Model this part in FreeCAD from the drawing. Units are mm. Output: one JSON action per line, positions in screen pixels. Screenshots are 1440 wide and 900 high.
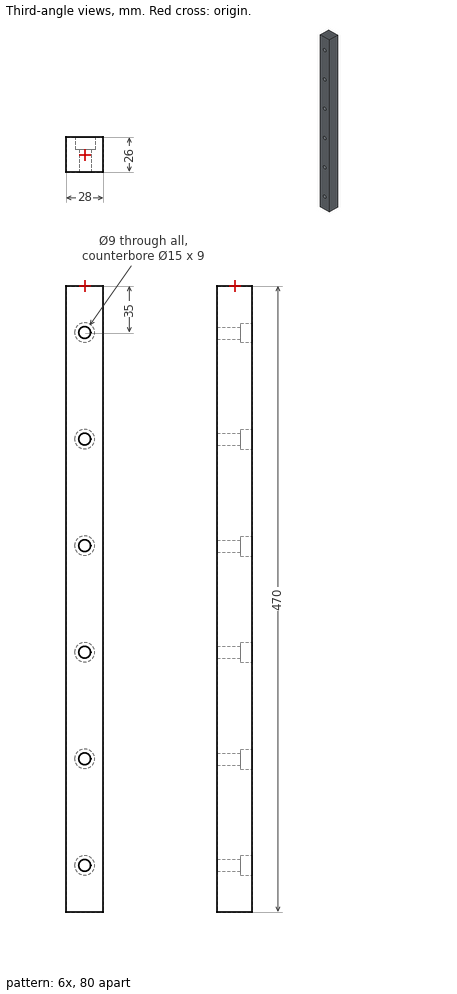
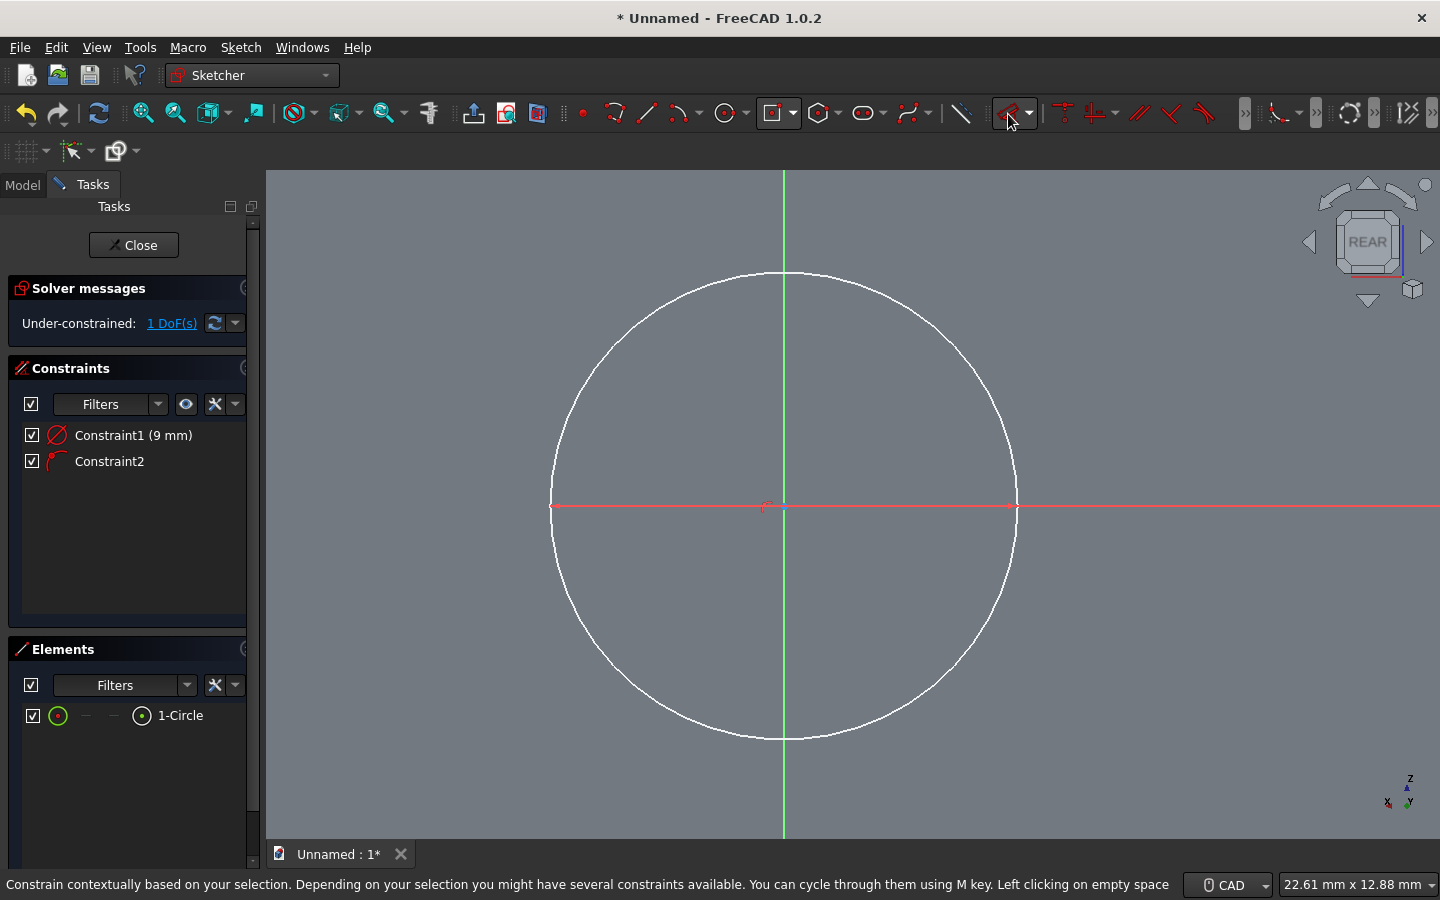
{"action": "left_click", "coordinate": [784, 506]}
{"action": "left_click", "coordinate": [818, 352]}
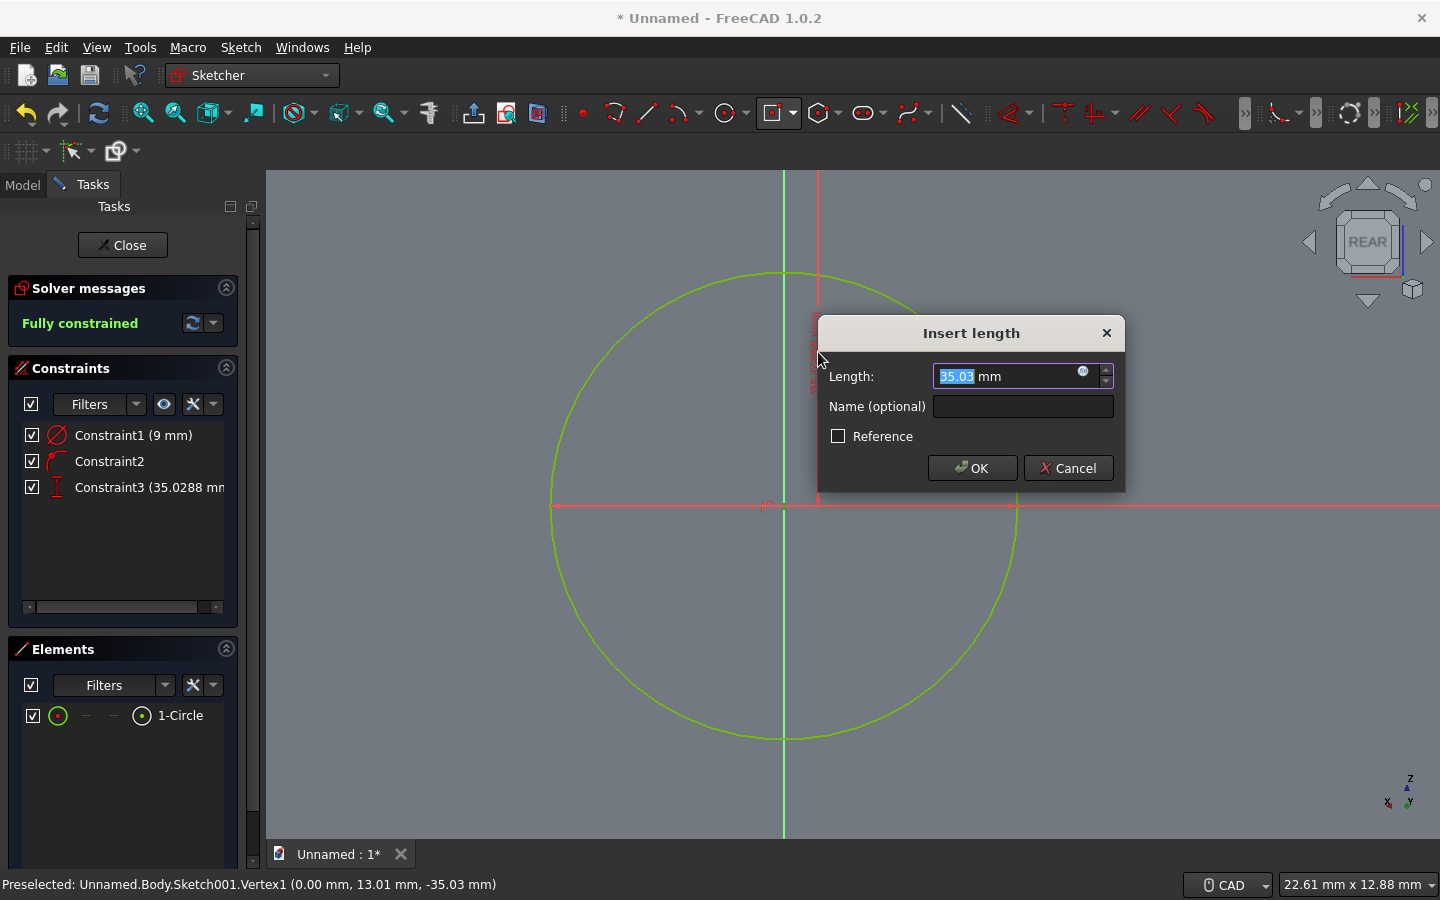
{"action": "type", "text": "35"}
{"action": "key", "text": "Return"}
{"action": "key", "text": "Escape"}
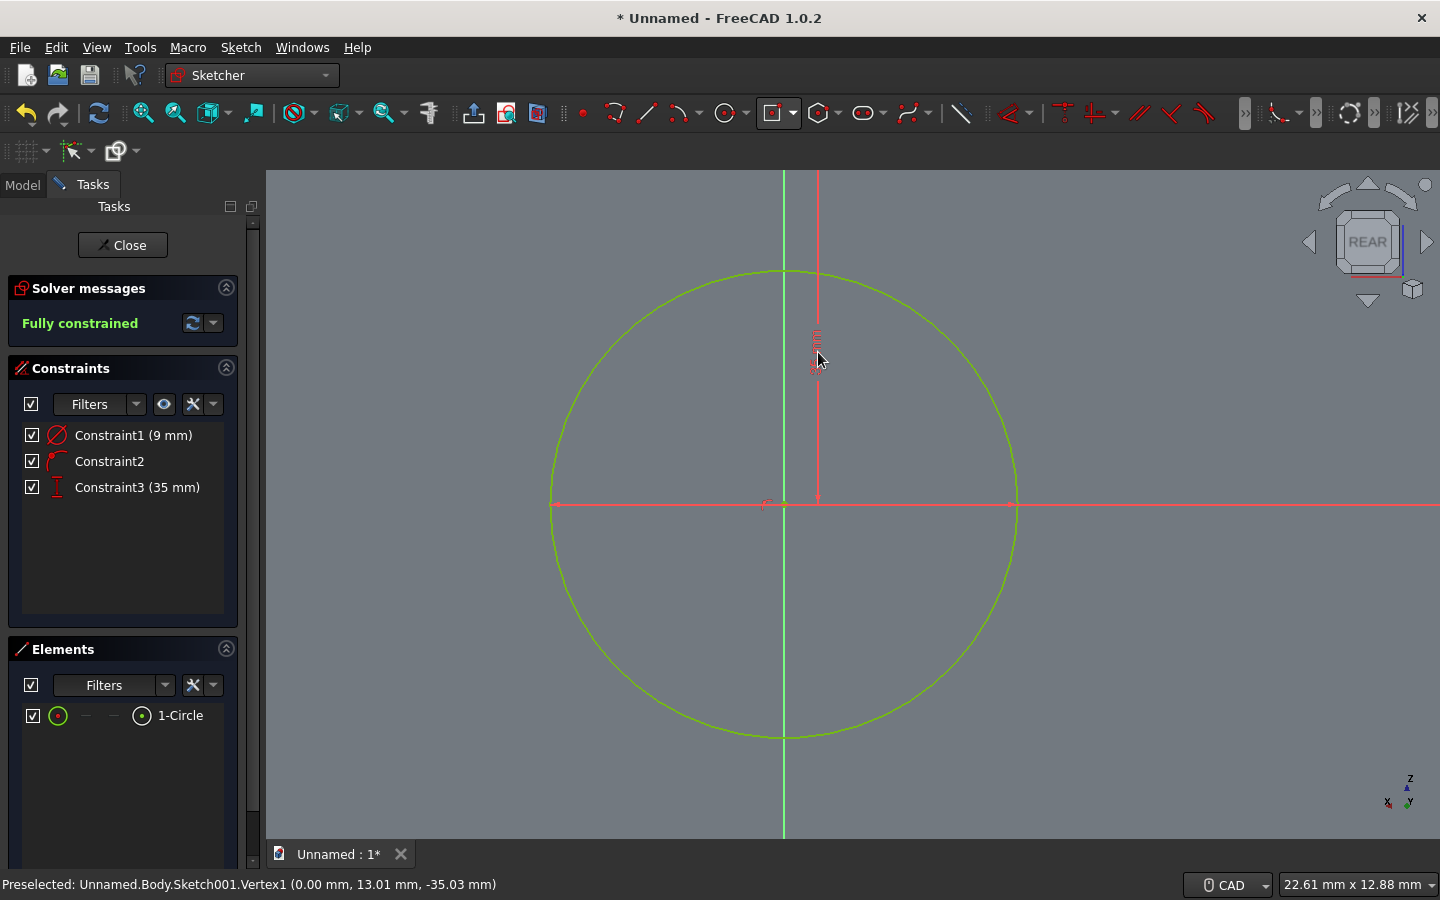
{"action": "left_click", "coordinate": [123, 245]}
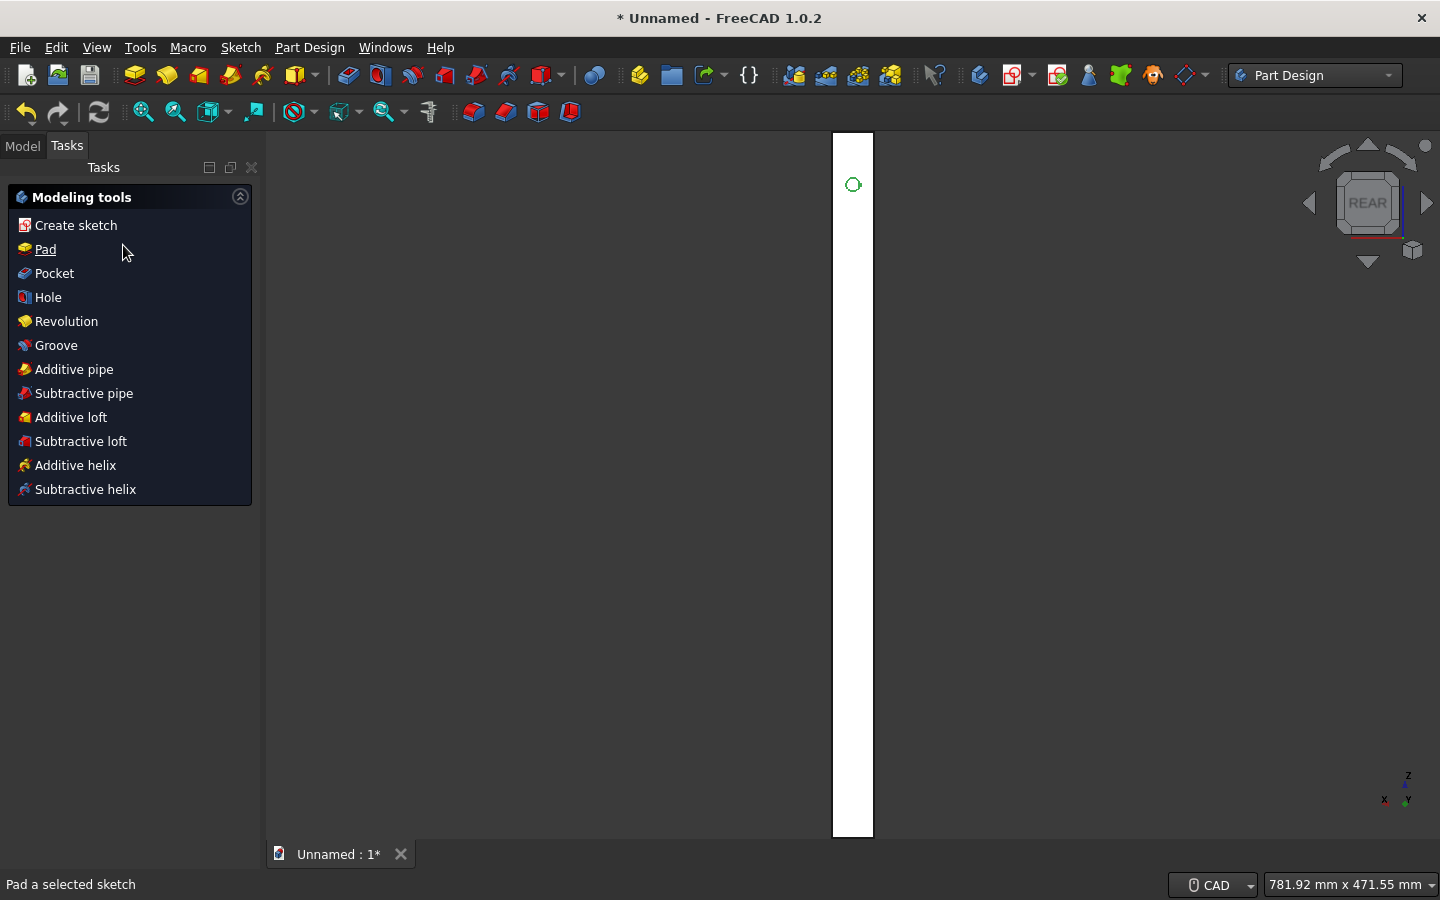
{"action": "left_click", "coordinate": [382, 76]}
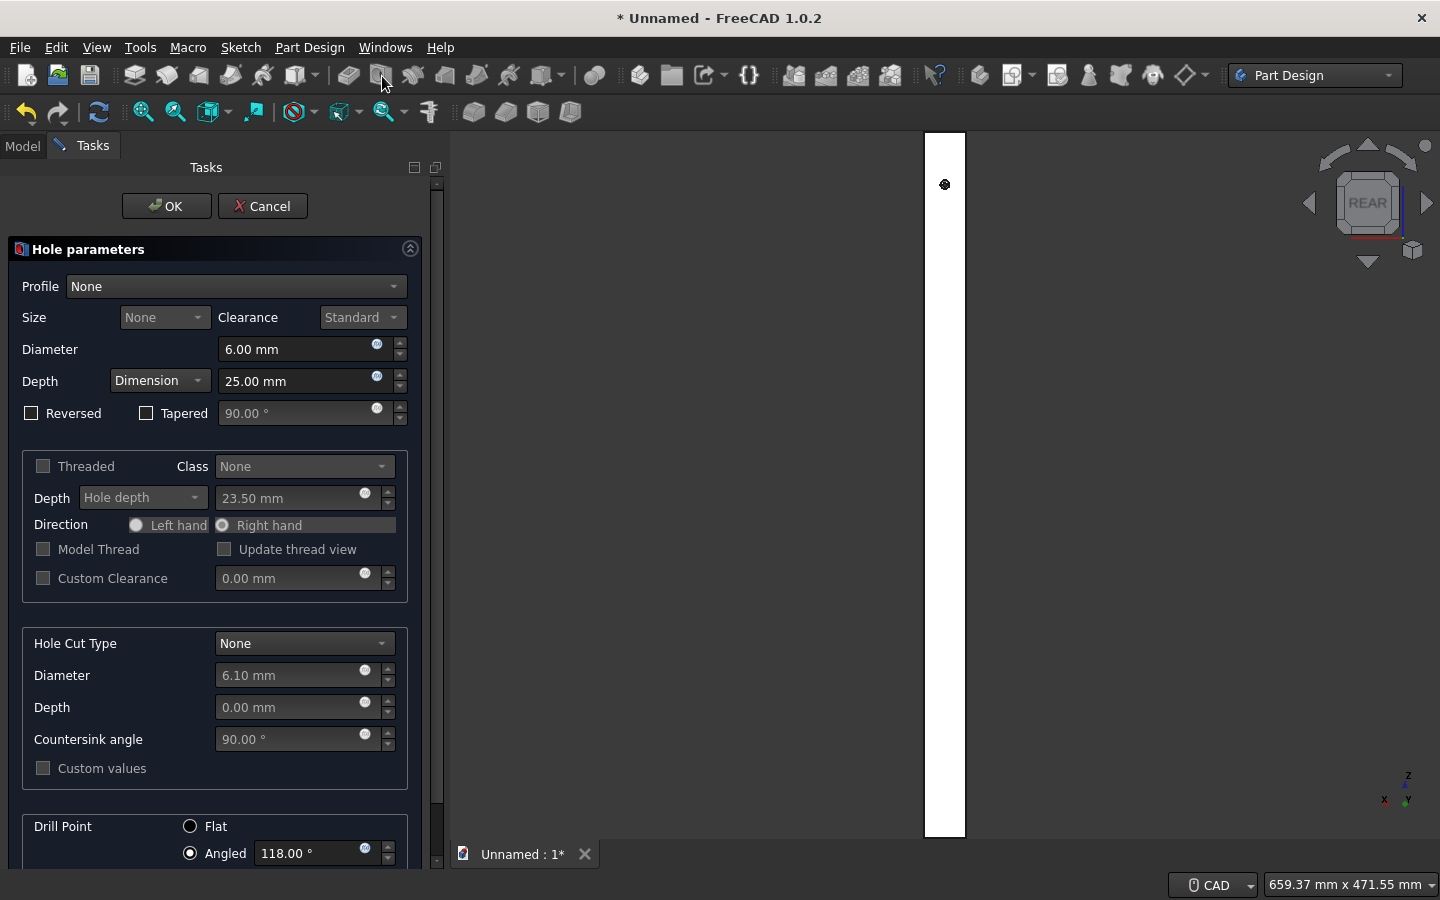
{"action": "triple_click", "coordinate": [305, 349]}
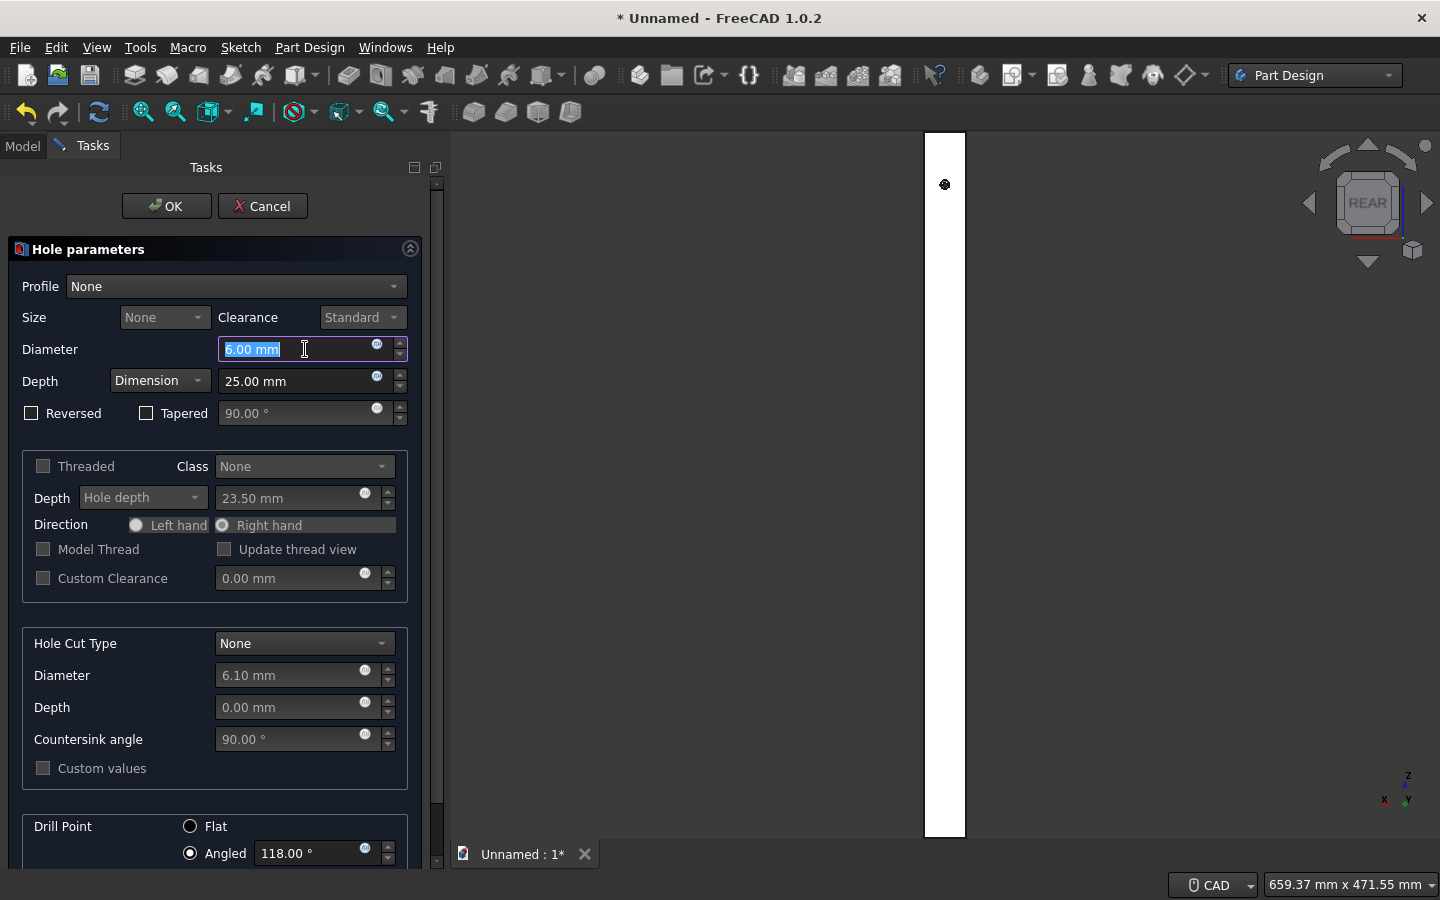
{"action": "type", "text": "9"}
{"action": "key", "text": "Tab"}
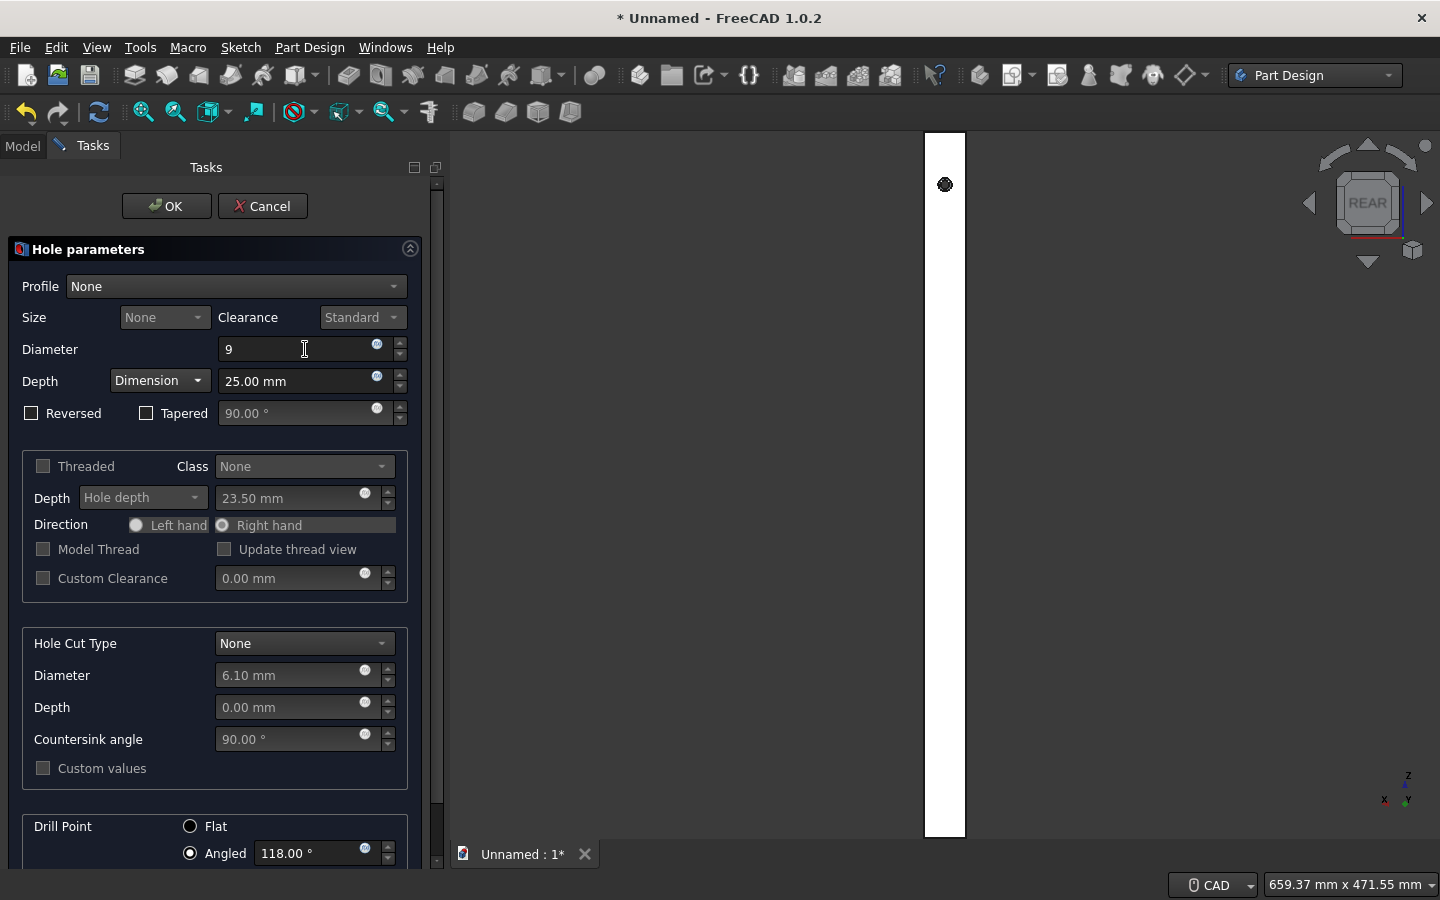
{"action": "left_click", "coordinate": [161, 380]}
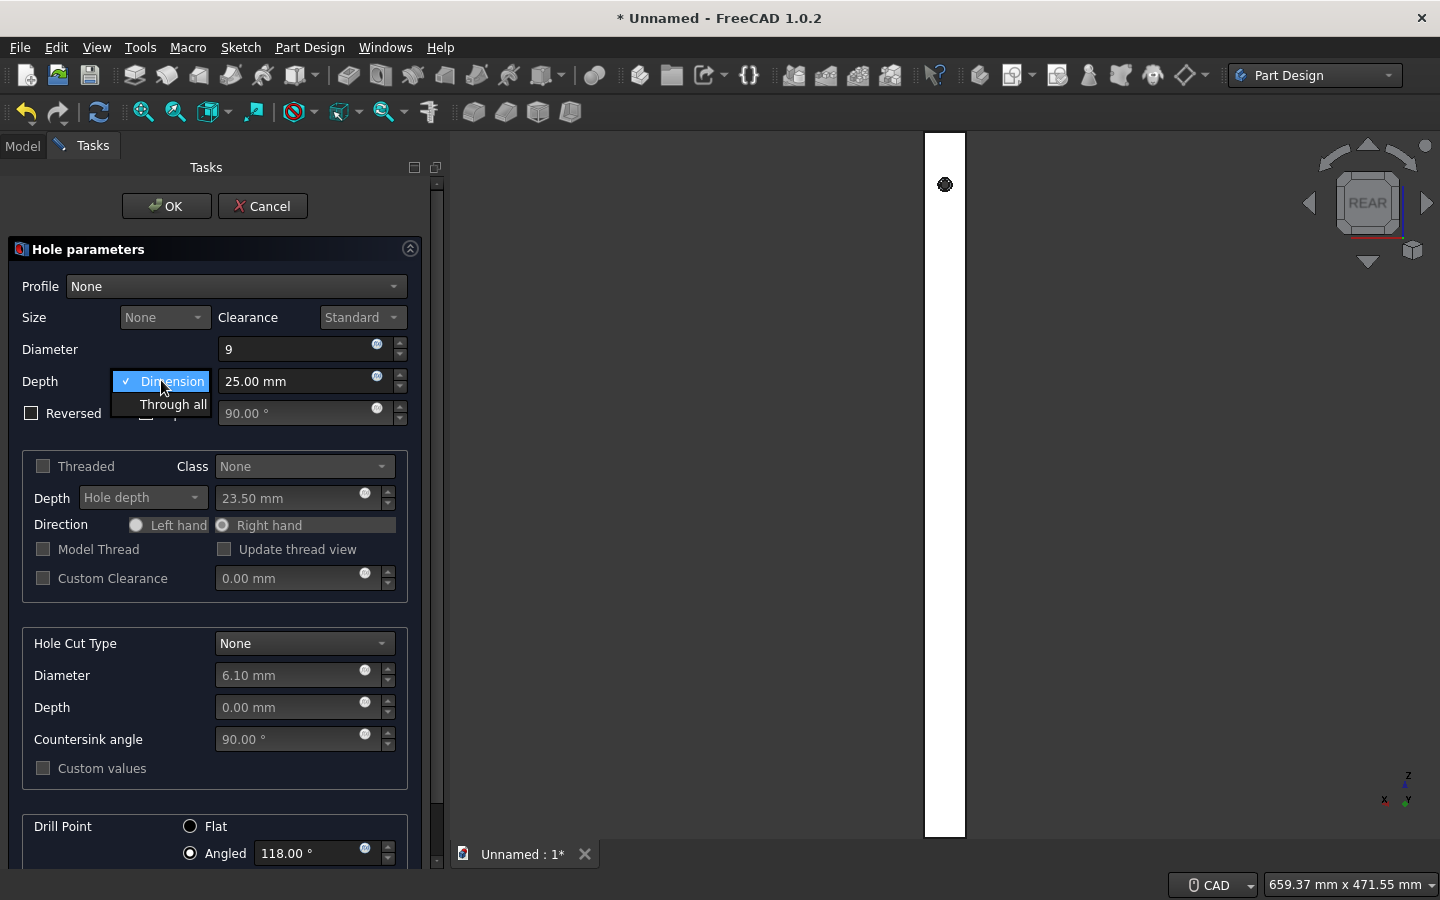
{"action": "left_click", "coordinate": [160, 404]}